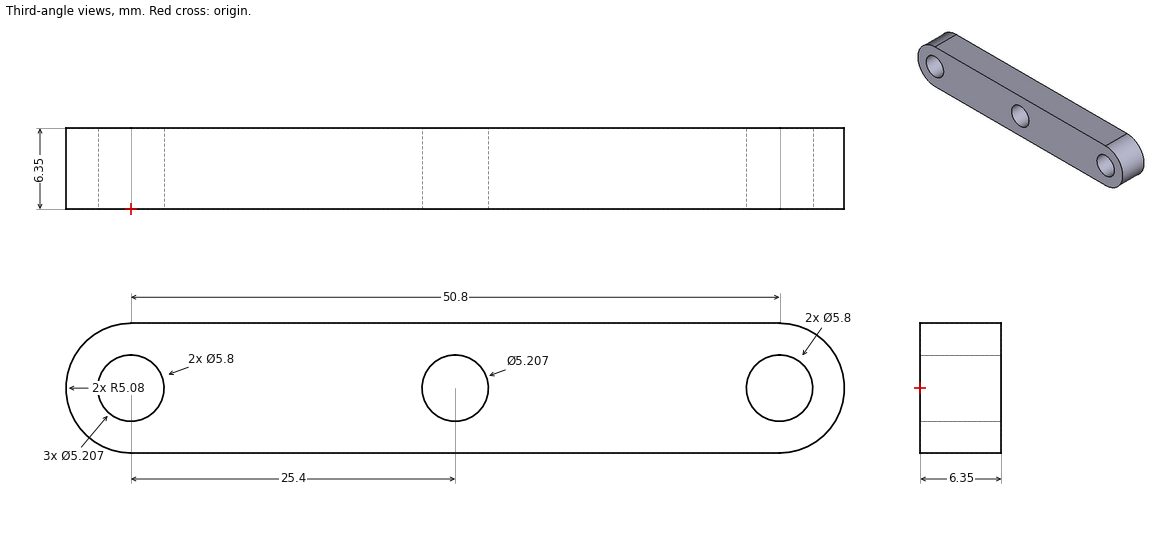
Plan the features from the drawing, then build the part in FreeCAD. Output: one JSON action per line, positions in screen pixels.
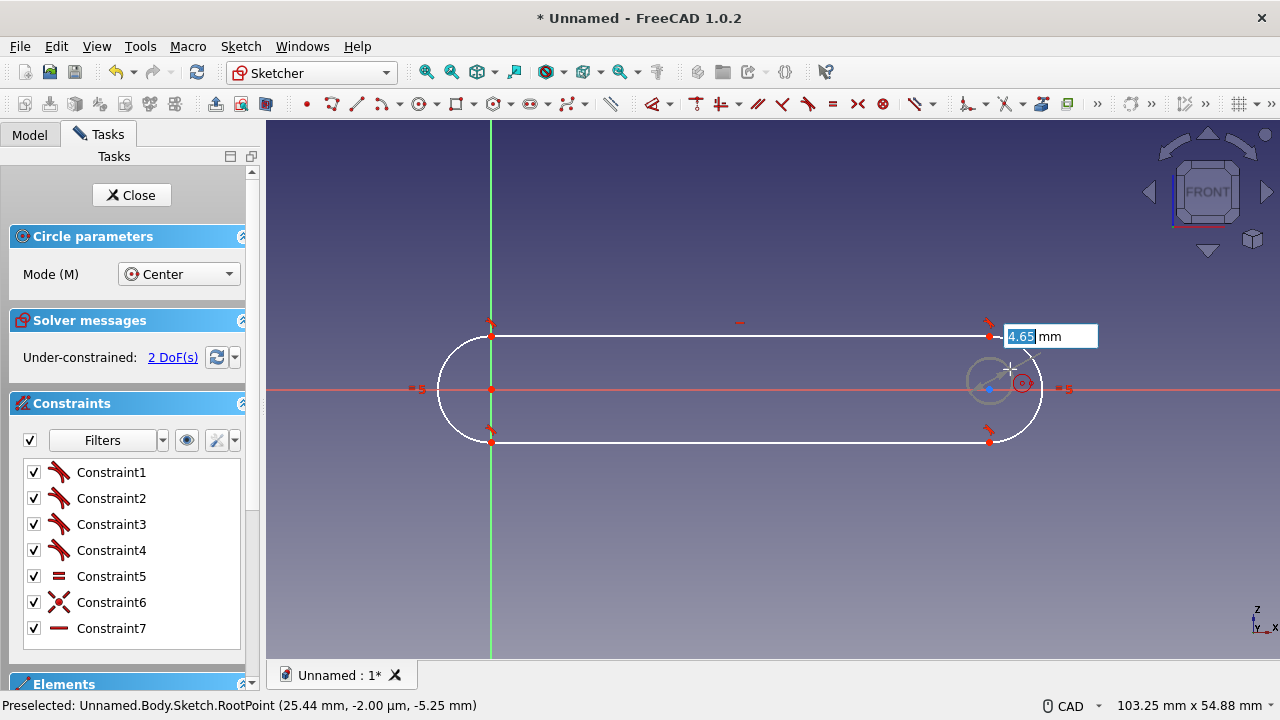
{"action": "type", "text": "5.8"}
{"action": "key", "text": "Return"}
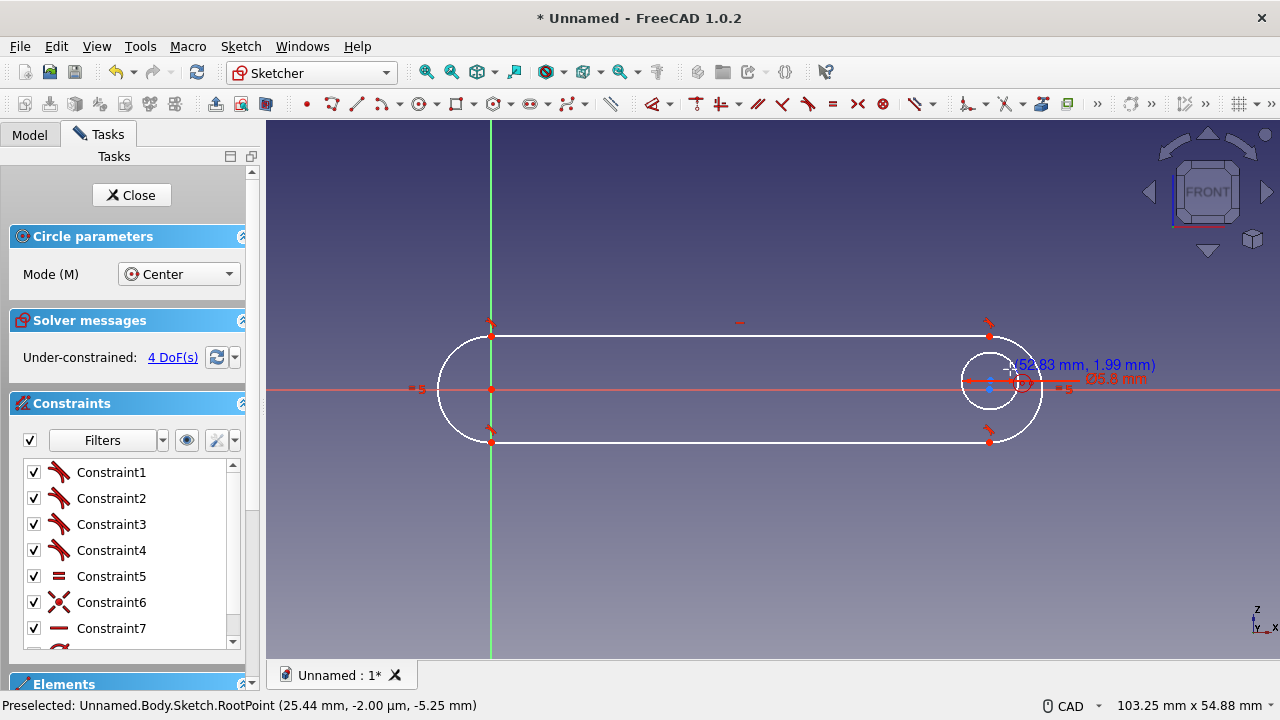
{"action": "left_click", "coordinate": [491, 390]}
{"action": "mouse_move", "coordinate": [511, 369]}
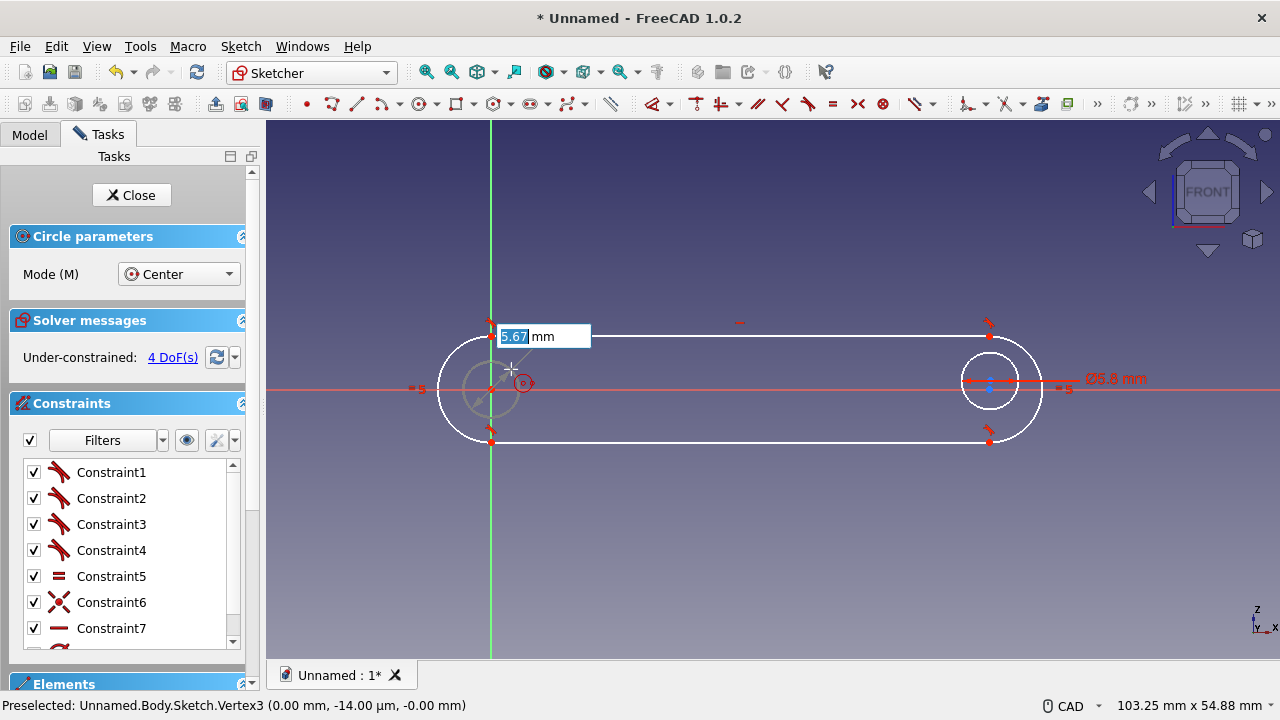
{"action": "type", "text": "5.8"}
{"action": "key", "text": "Return"}
{"action": "key", "text": "Escape"}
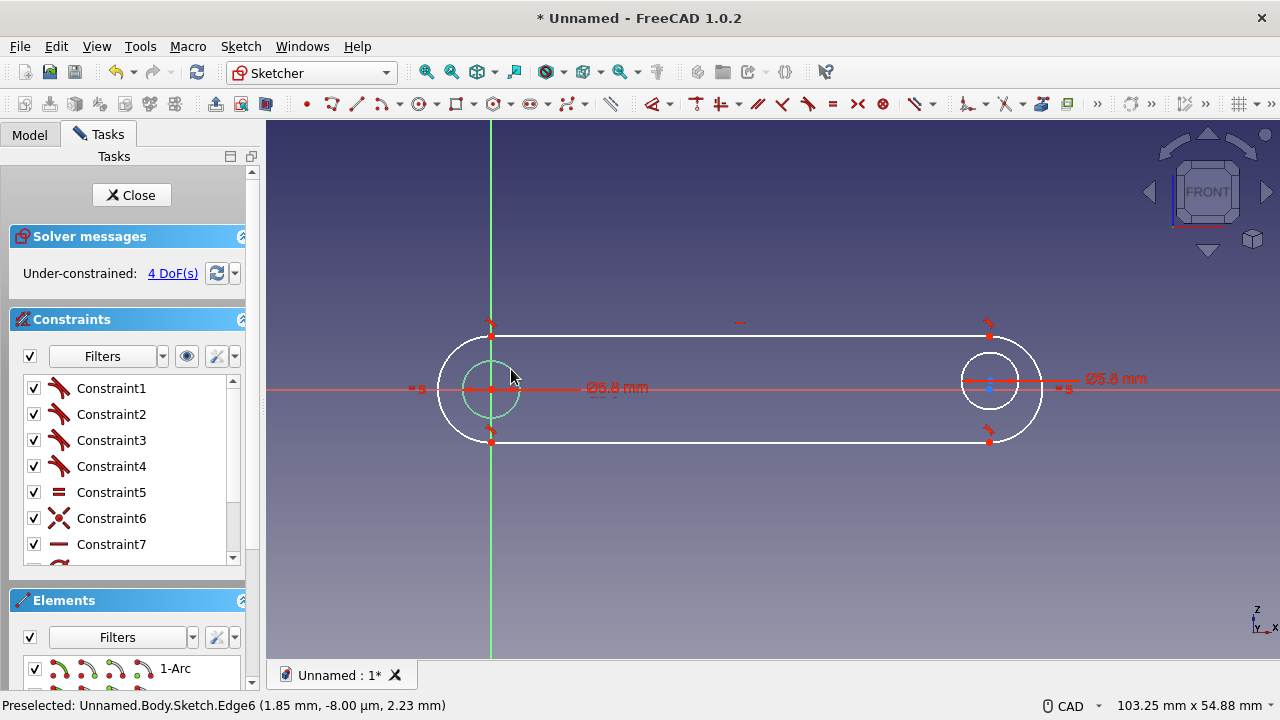
{"action": "left_click", "coordinate": [1010, 361]}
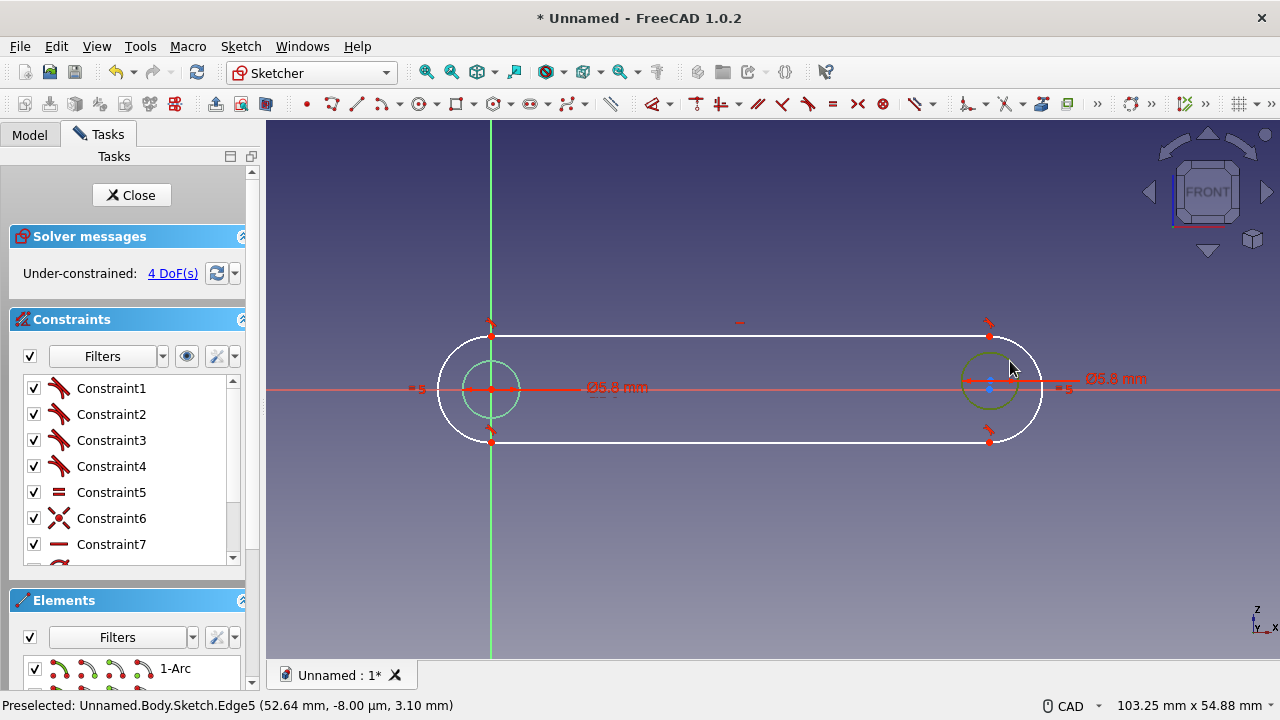
{"action": "left_click", "coordinate": [1032, 421]}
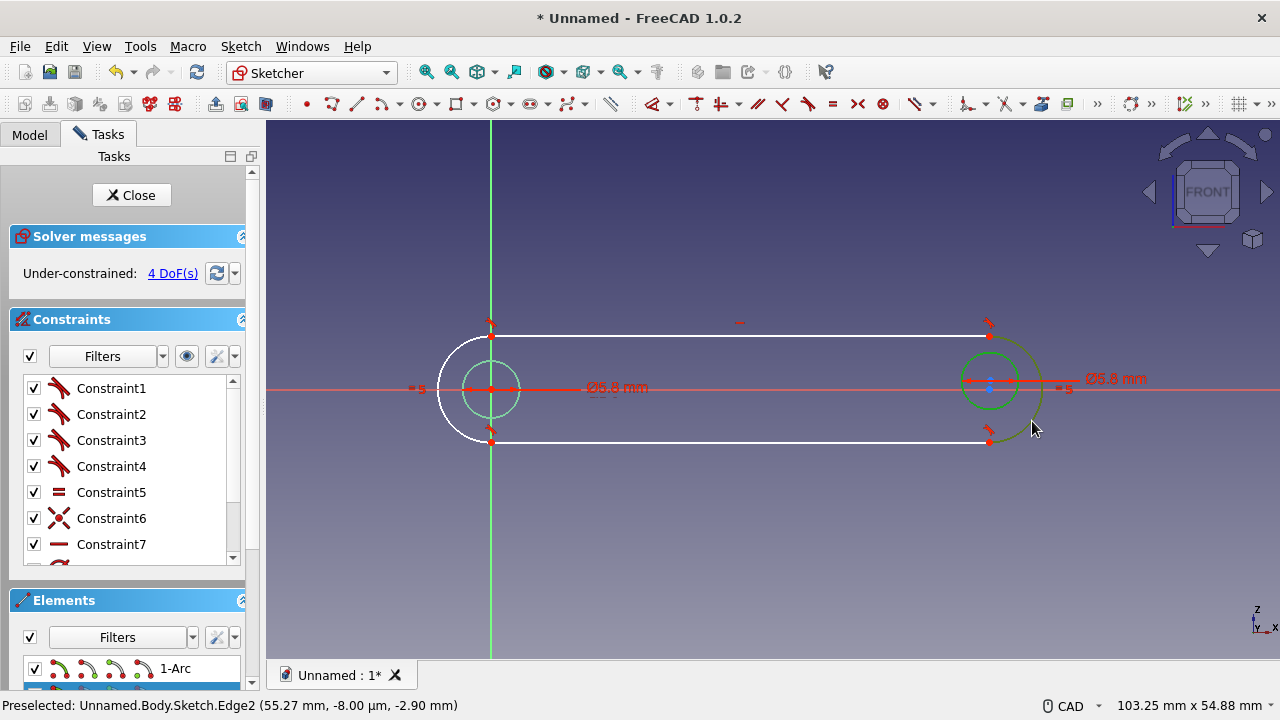
{"action": "left_click", "coordinate": [696, 104]}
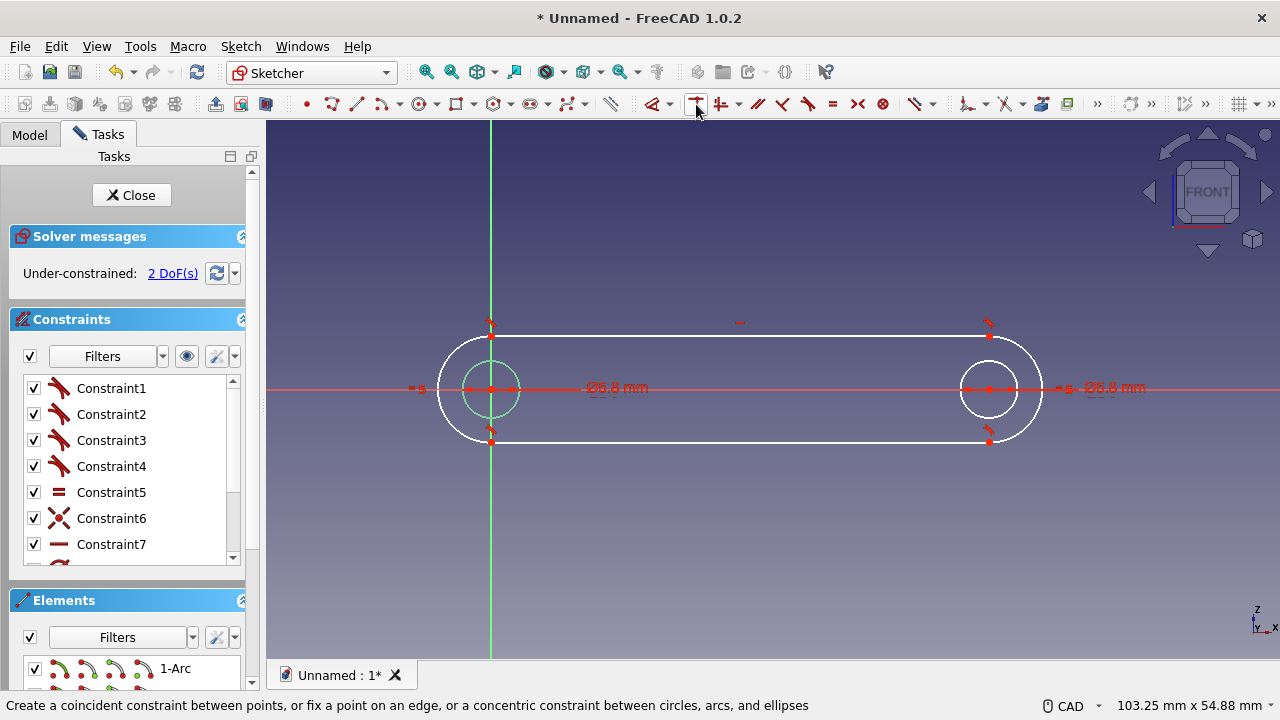
{"action": "left_click", "coordinate": [652, 104]}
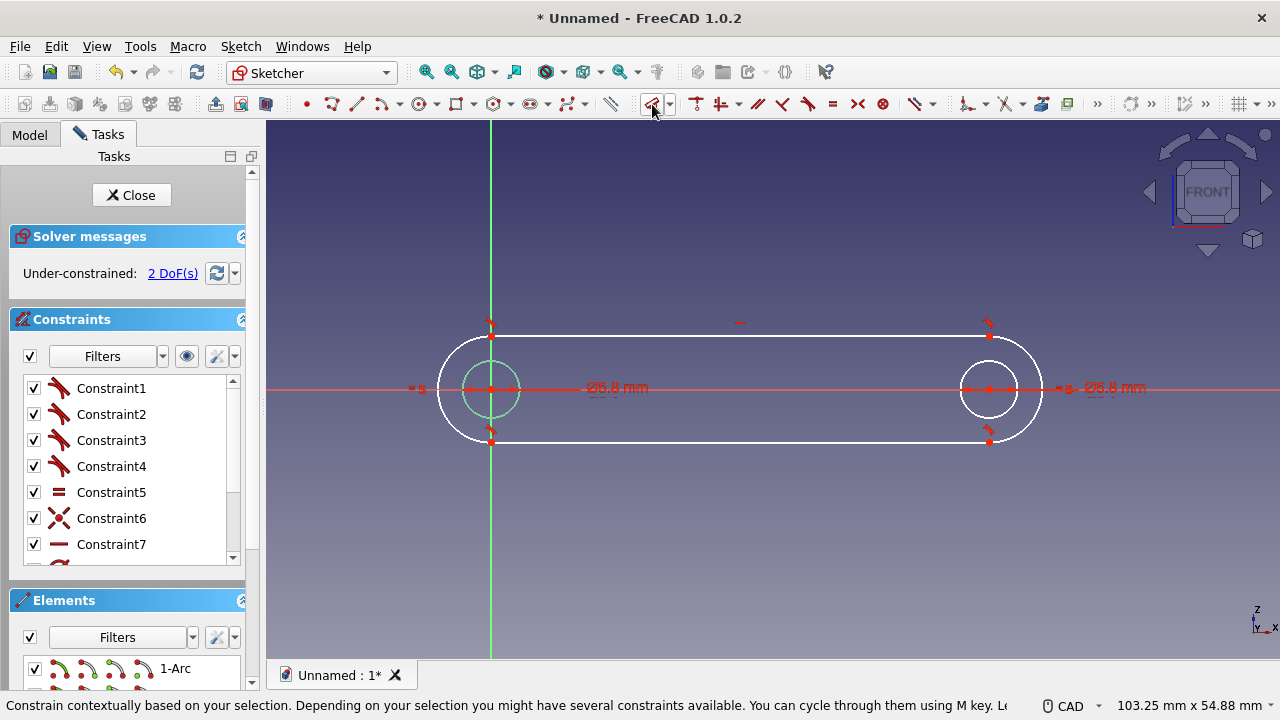
{"action": "left_click", "coordinate": [448, 358]}
{"action": "left_click", "coordinate": [422, 339]}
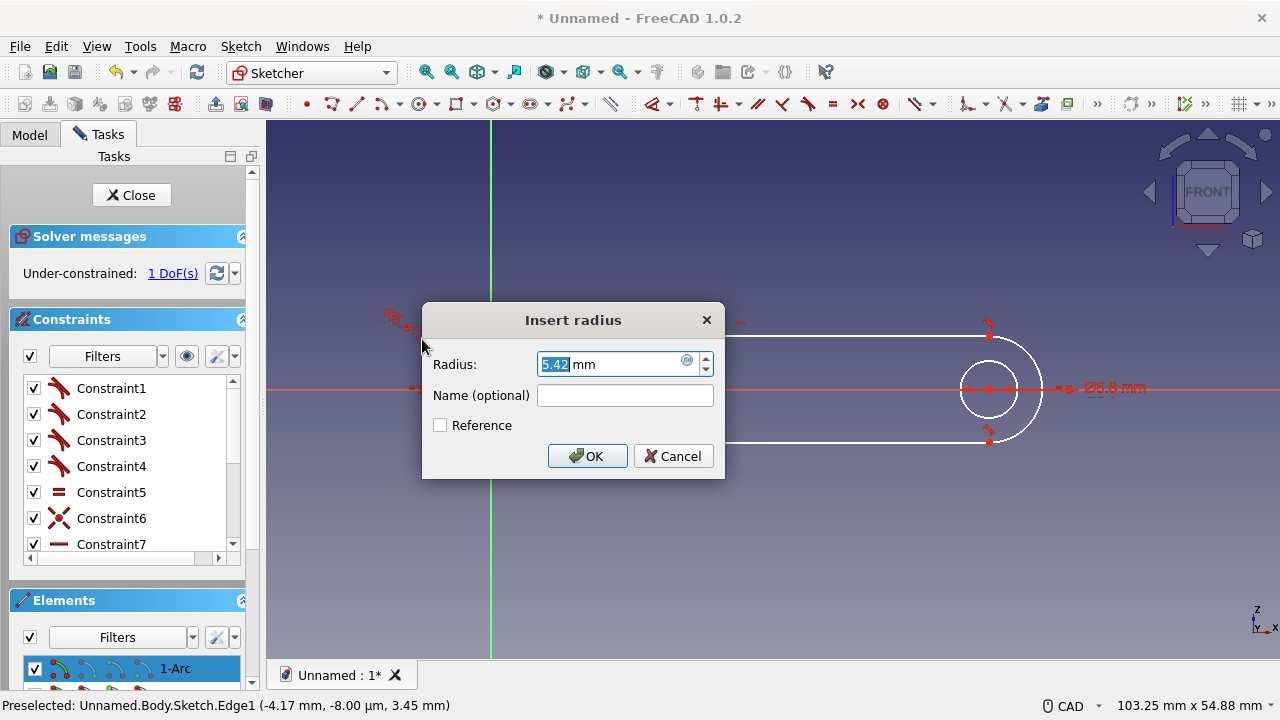
{"action": "type", "text": "5.08"}
{"action": "key", "text": "Return"}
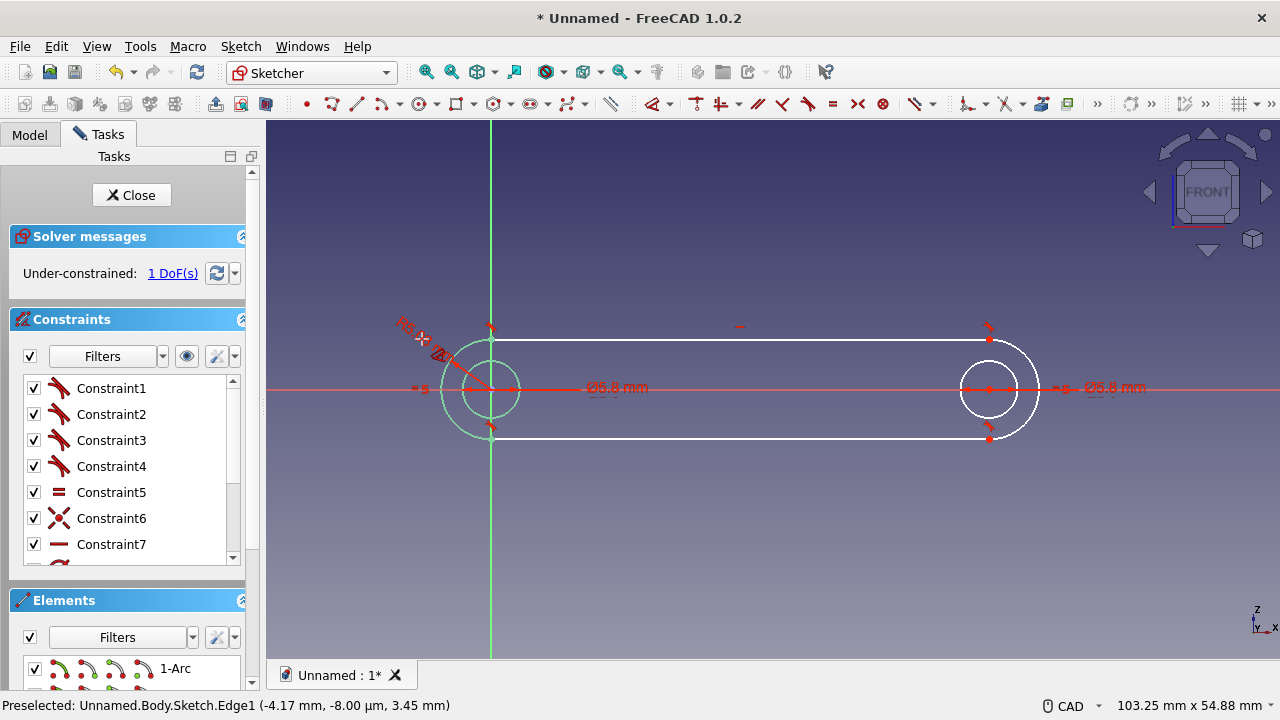
{"action": "left_click", "coordinate": [641, 340]}
{"action": "left_click", "coordinate": [740, 306]}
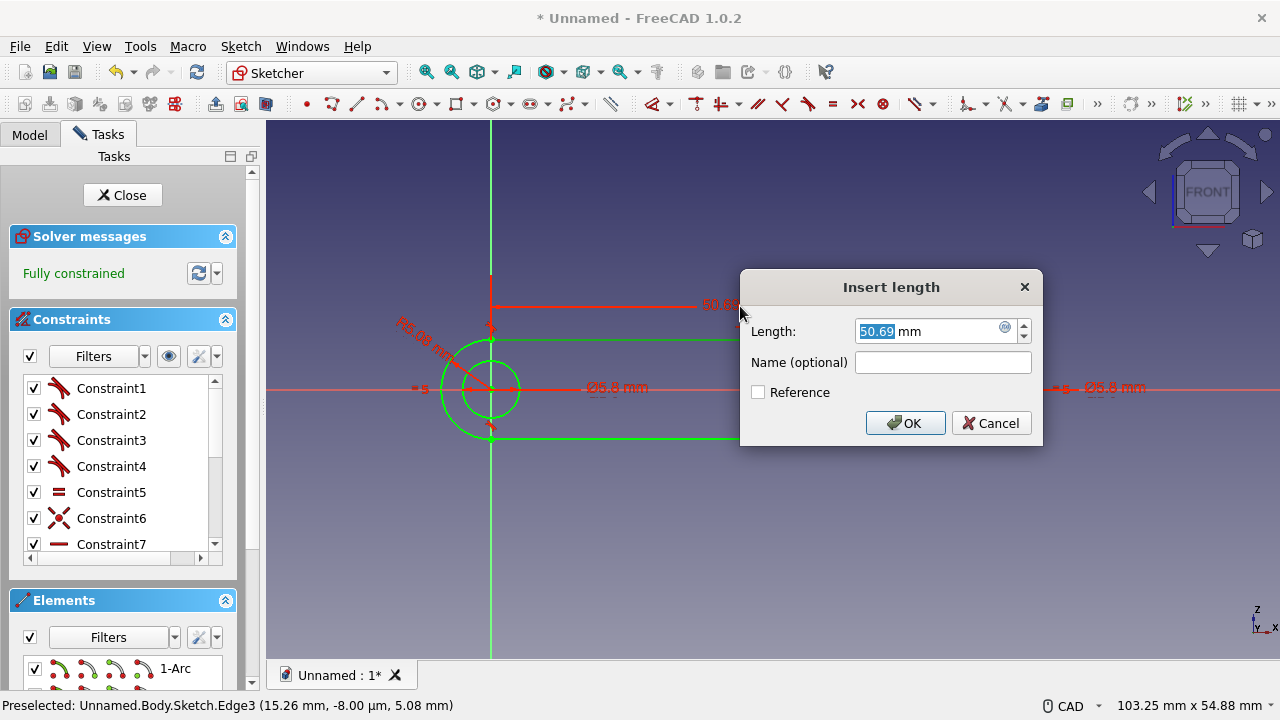
{"action": "type", "text": "50.8"}
{"action": "key", "text": "Return"}
{"action": "key", "text": "Escape"}